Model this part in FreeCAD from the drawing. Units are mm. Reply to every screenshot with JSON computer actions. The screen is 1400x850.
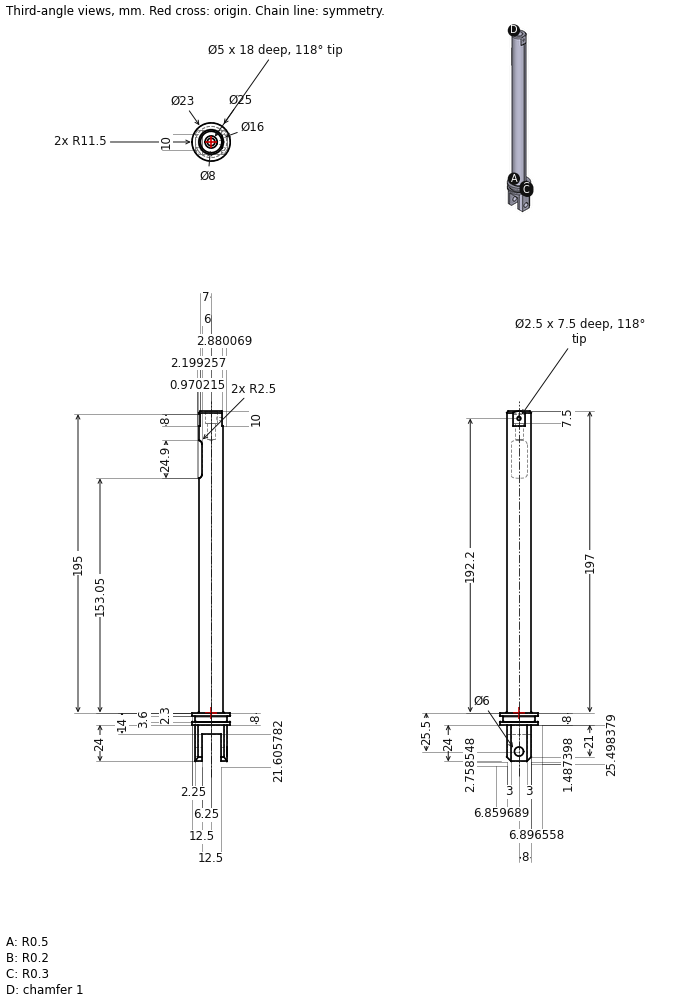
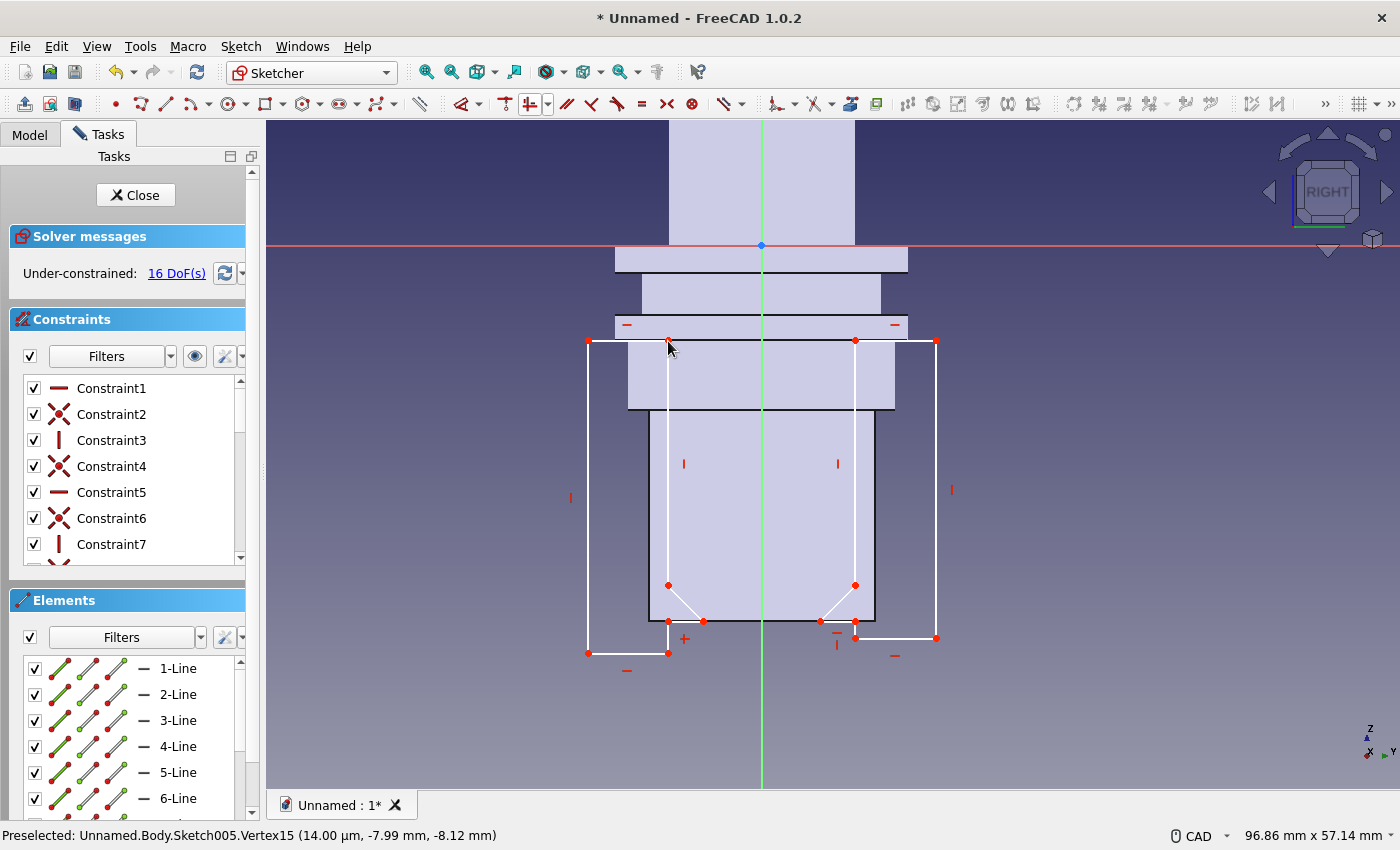
{"action": "left_click", "coordinate": [855, 341]}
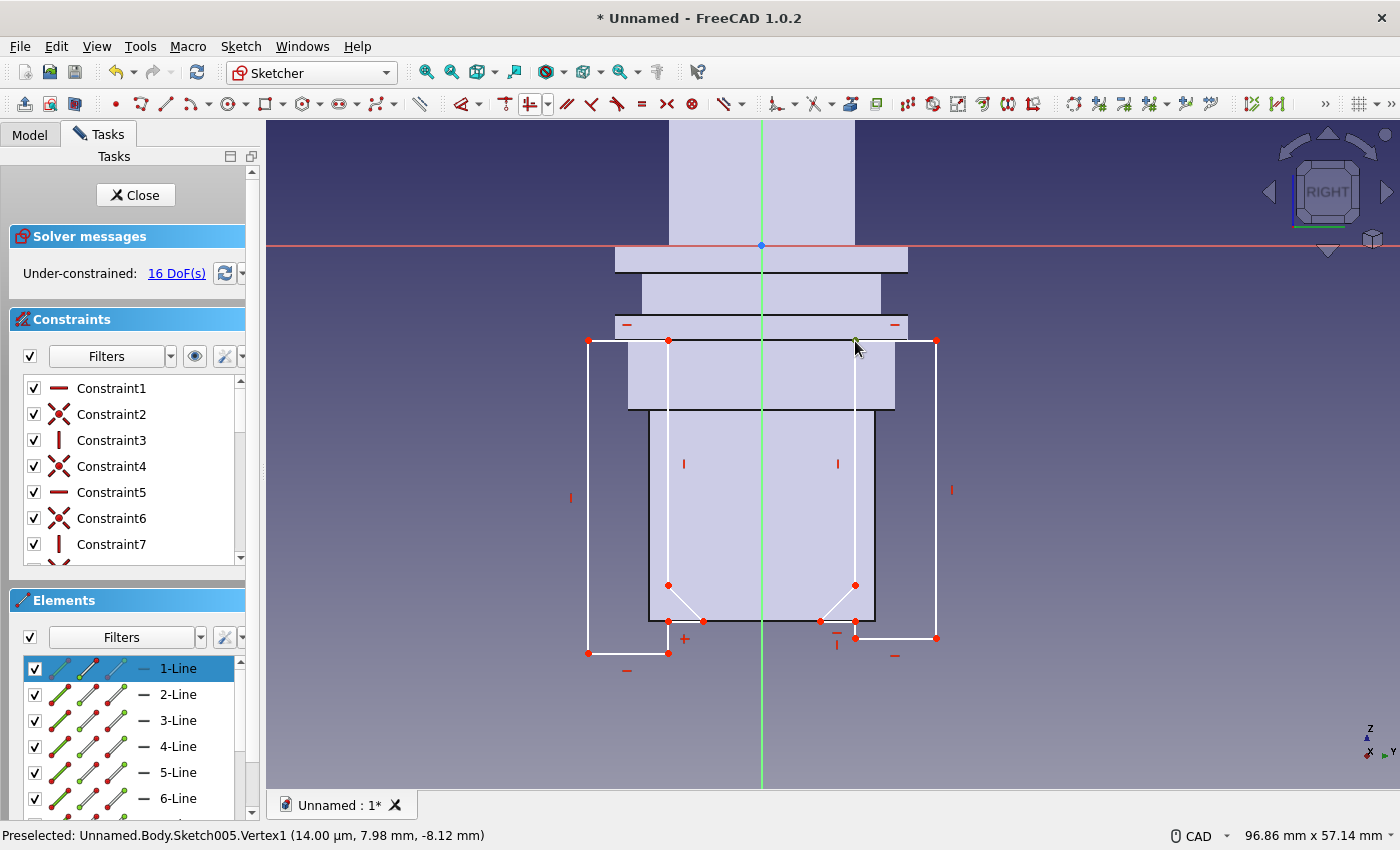
{"action": "left_click", "coordinate": [668, 341]}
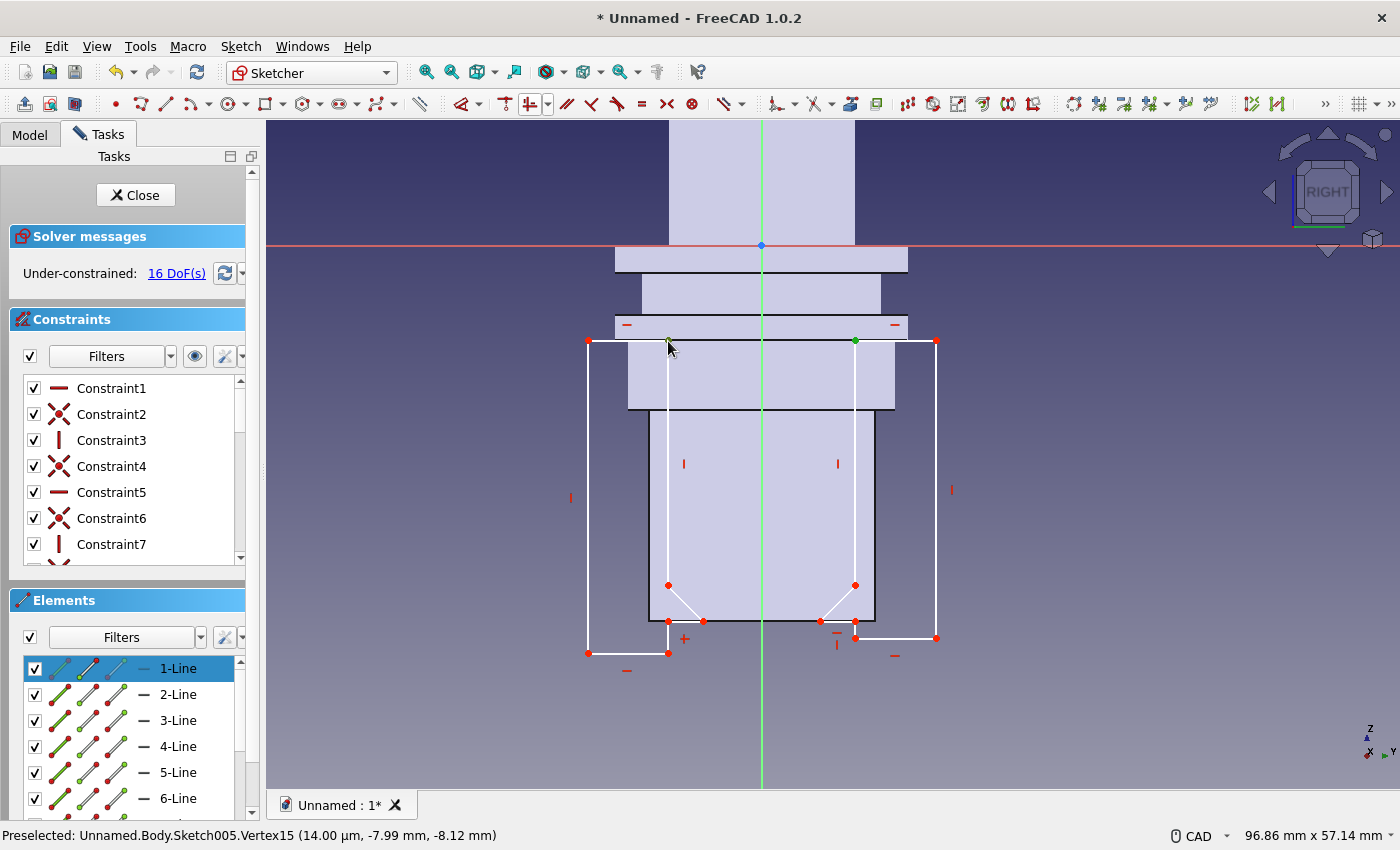
{"action": "left_click", "coordinate": [762, 717]}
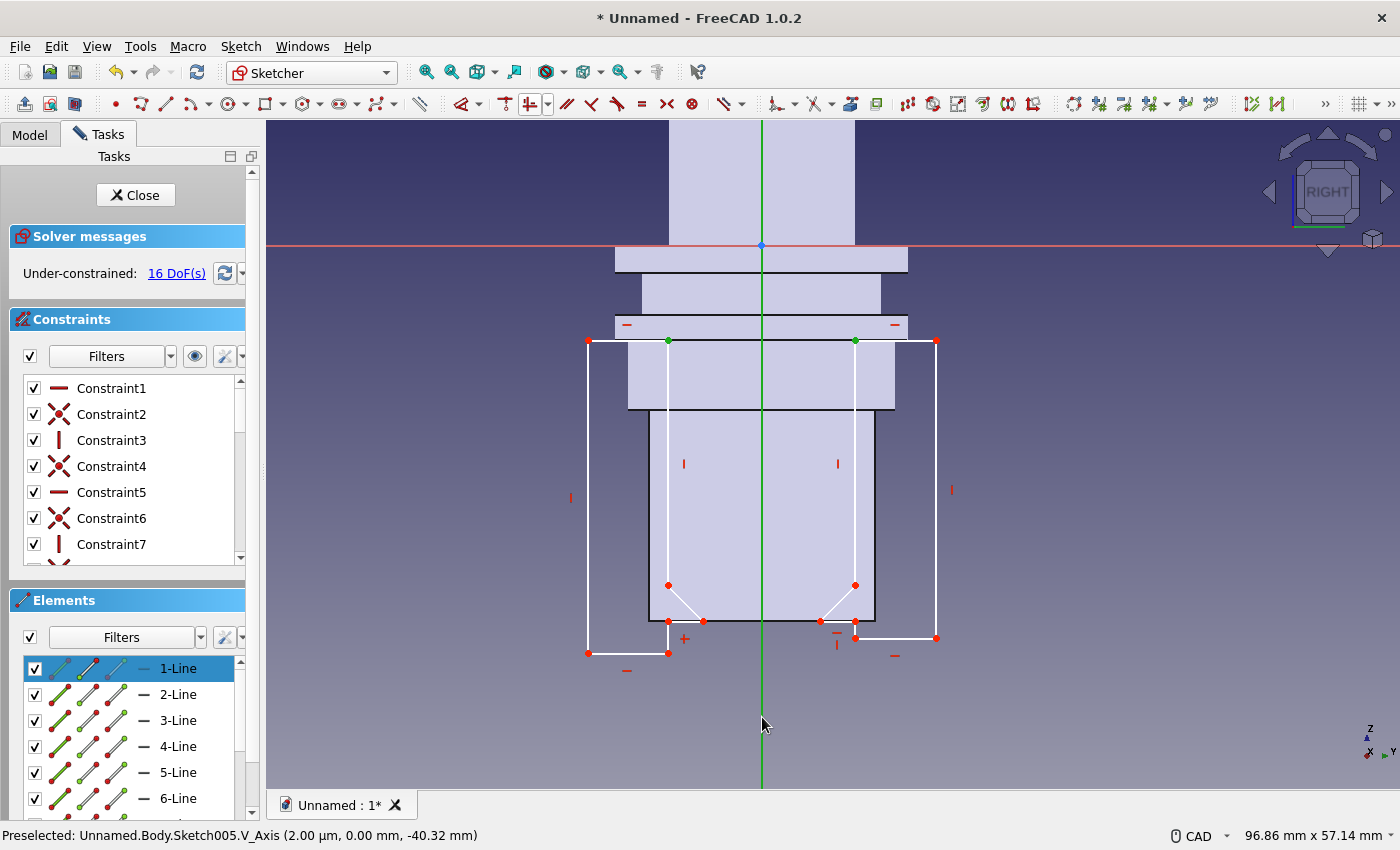
{"action": "left_click", "coordinate": [667, 104]}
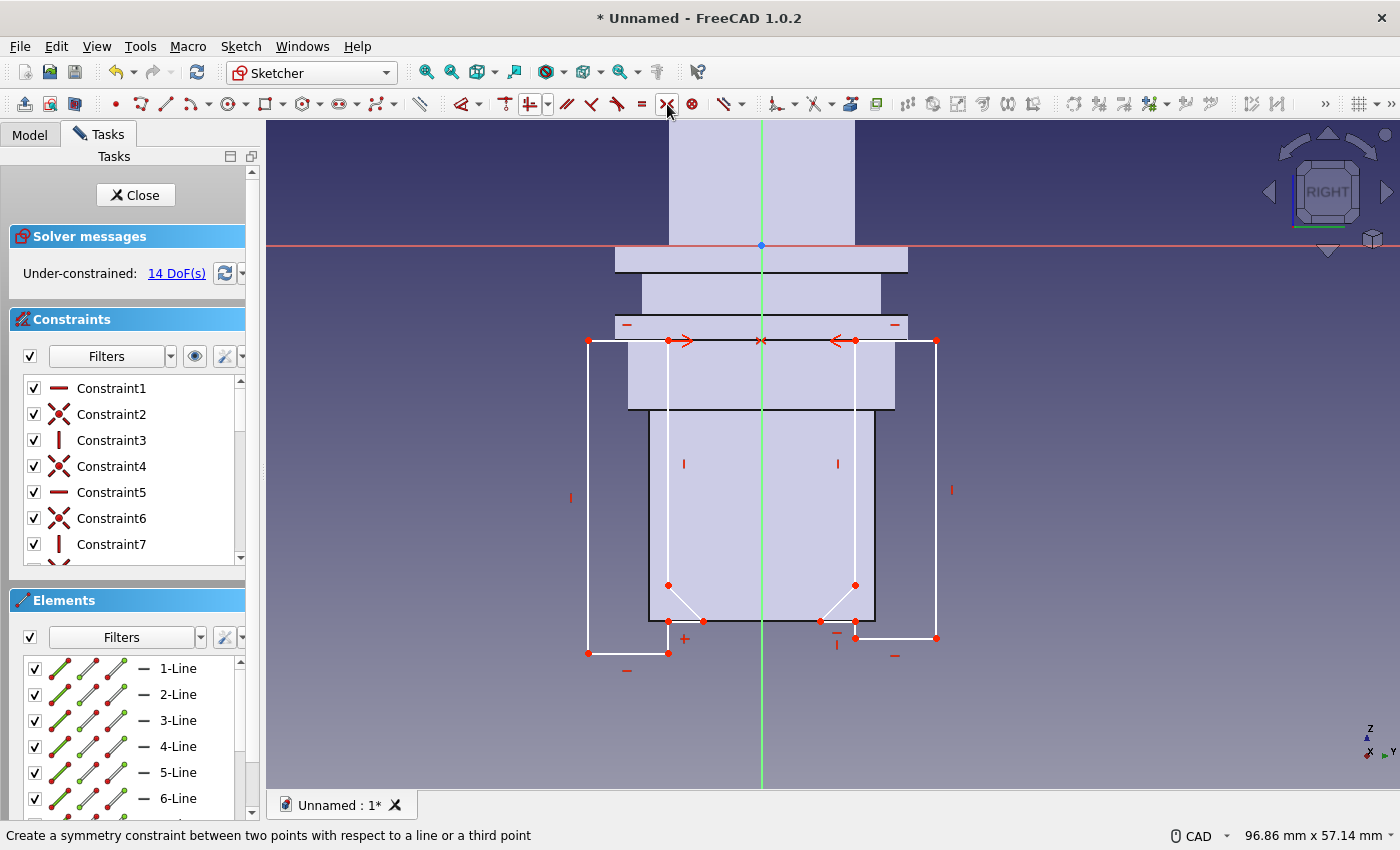
{"action": "left_click", "coordinate": [820, 622]}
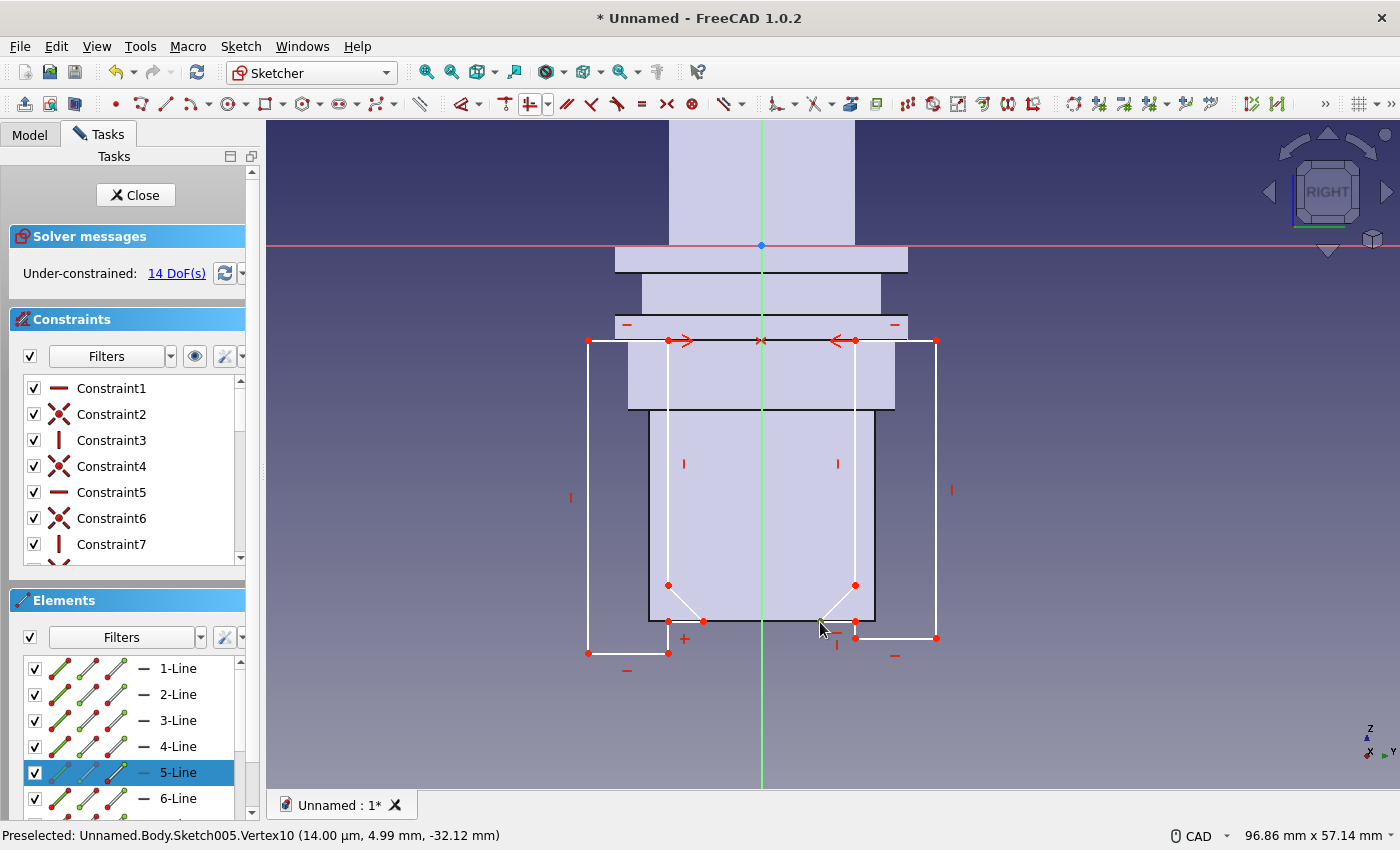
{"action": "left_click", "coordinate": [703, 622]}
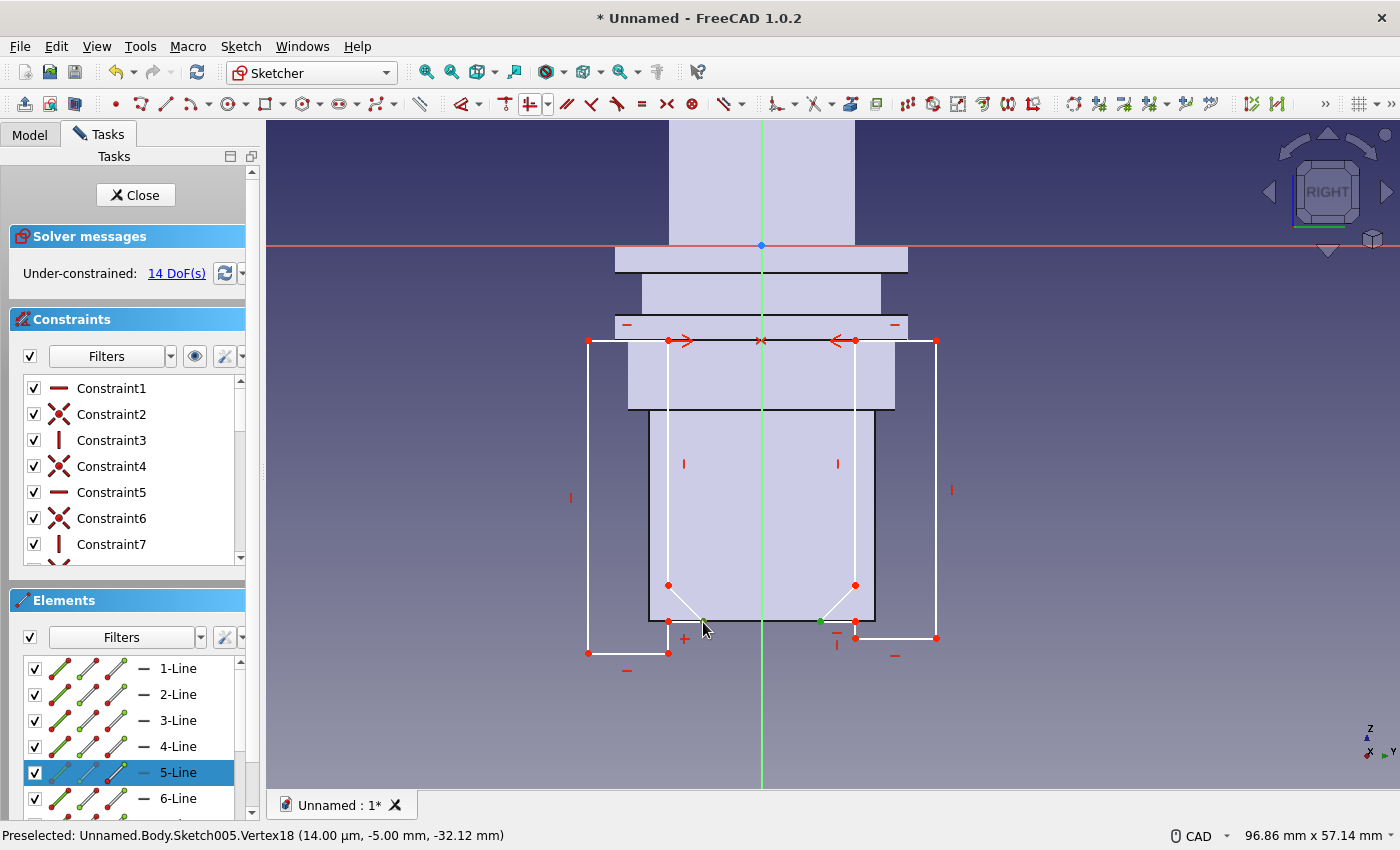
{"action": "left_click", "coordinate": [762, 717]}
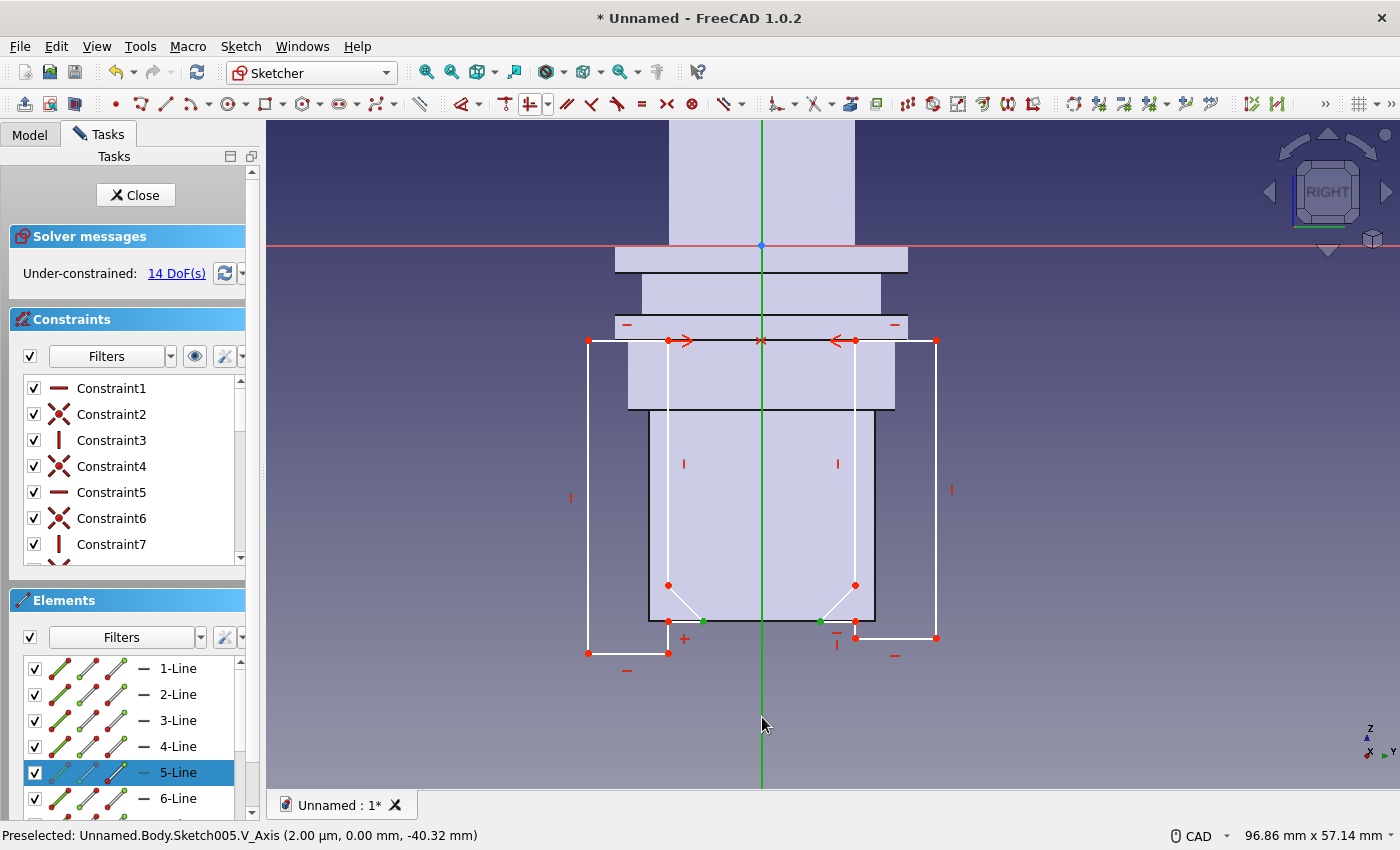
{"action": "left_click", "coordinate": [667, 104]}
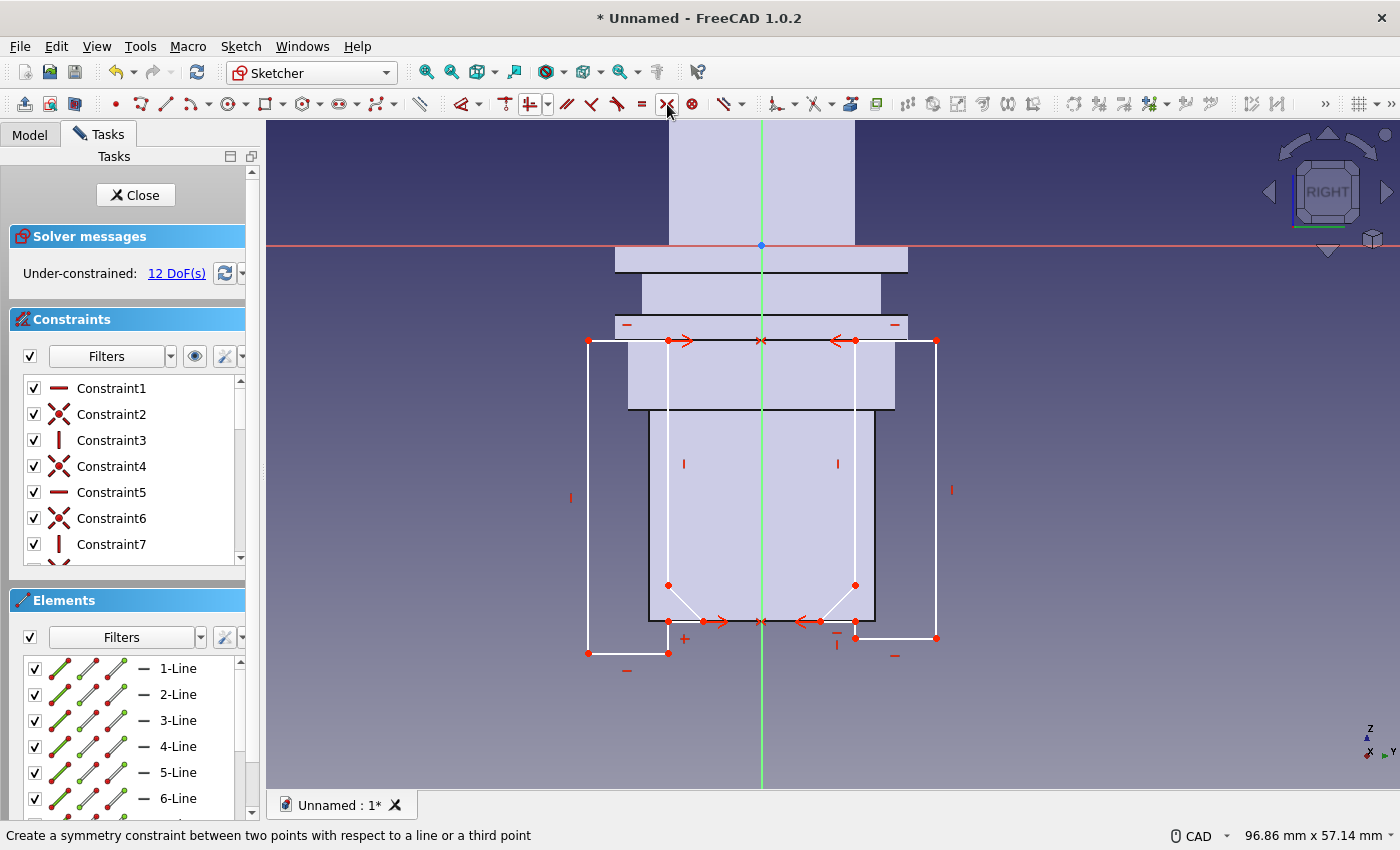
{"action": "left_click", "coordinate": [460, 104]}